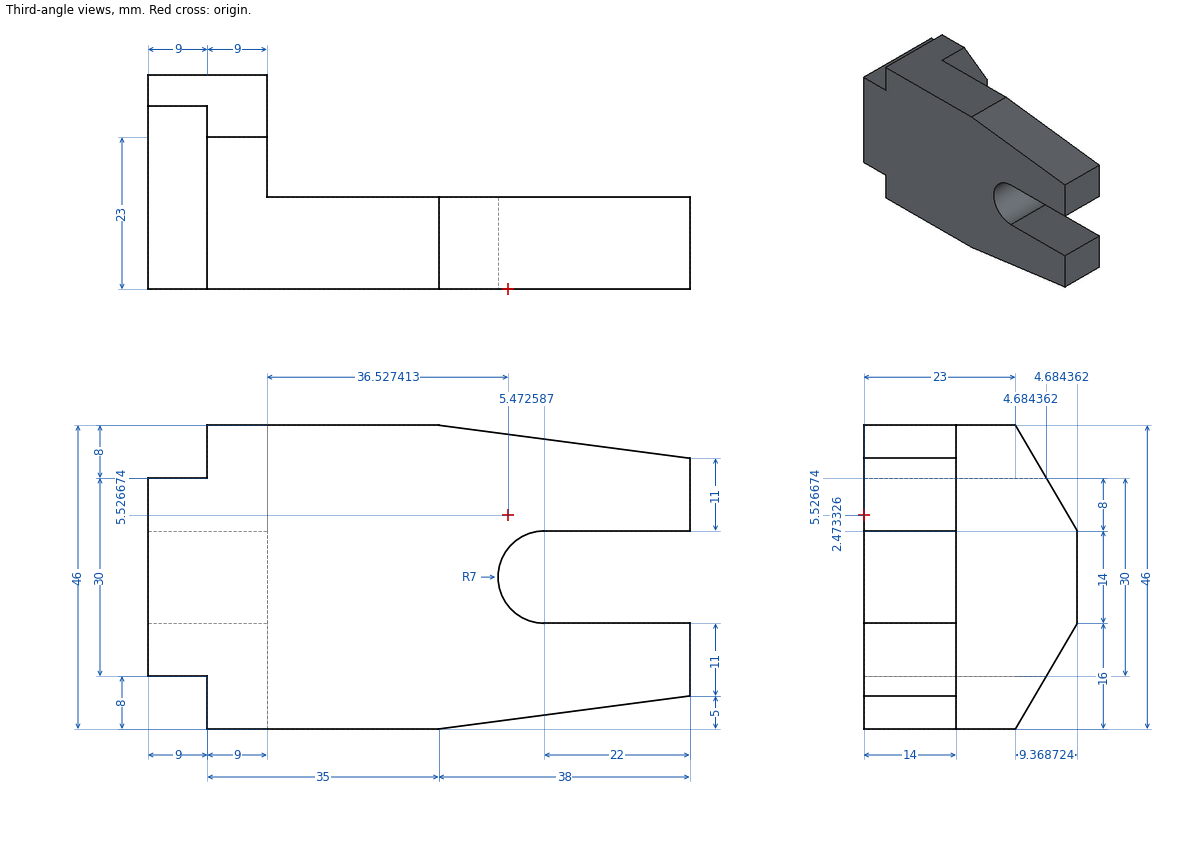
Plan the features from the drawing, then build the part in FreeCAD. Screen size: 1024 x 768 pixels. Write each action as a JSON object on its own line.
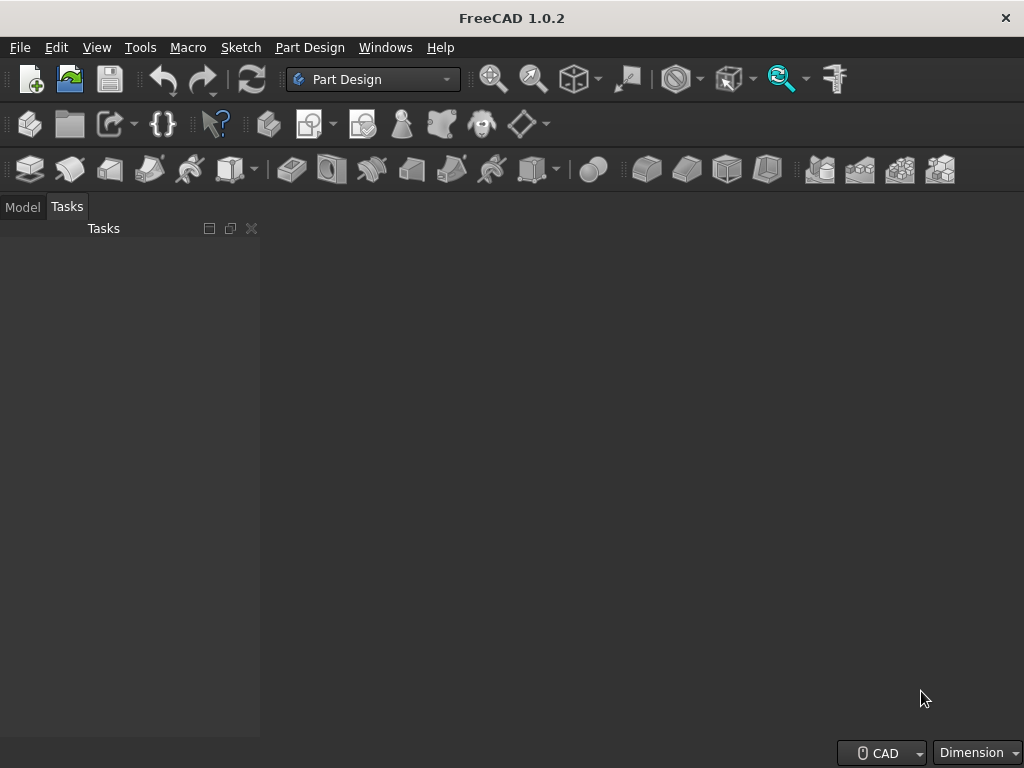
{"action": "left_click", "coordinate": [30, 80]}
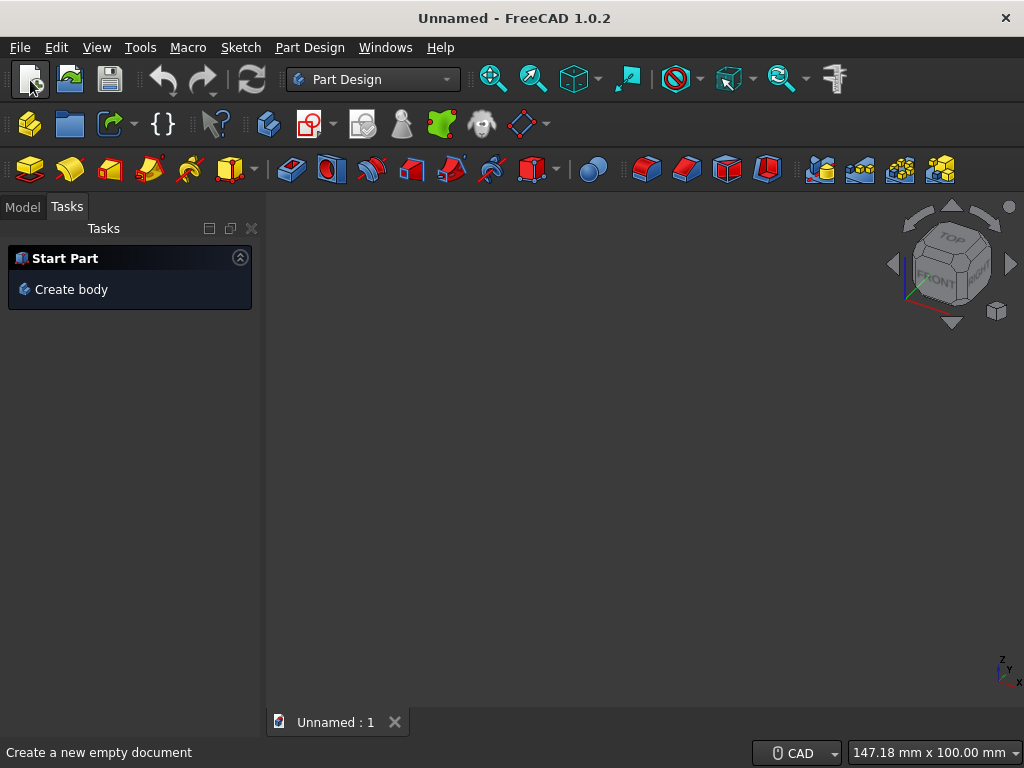
{"action": "left_click", "coordinate": [310, 124]}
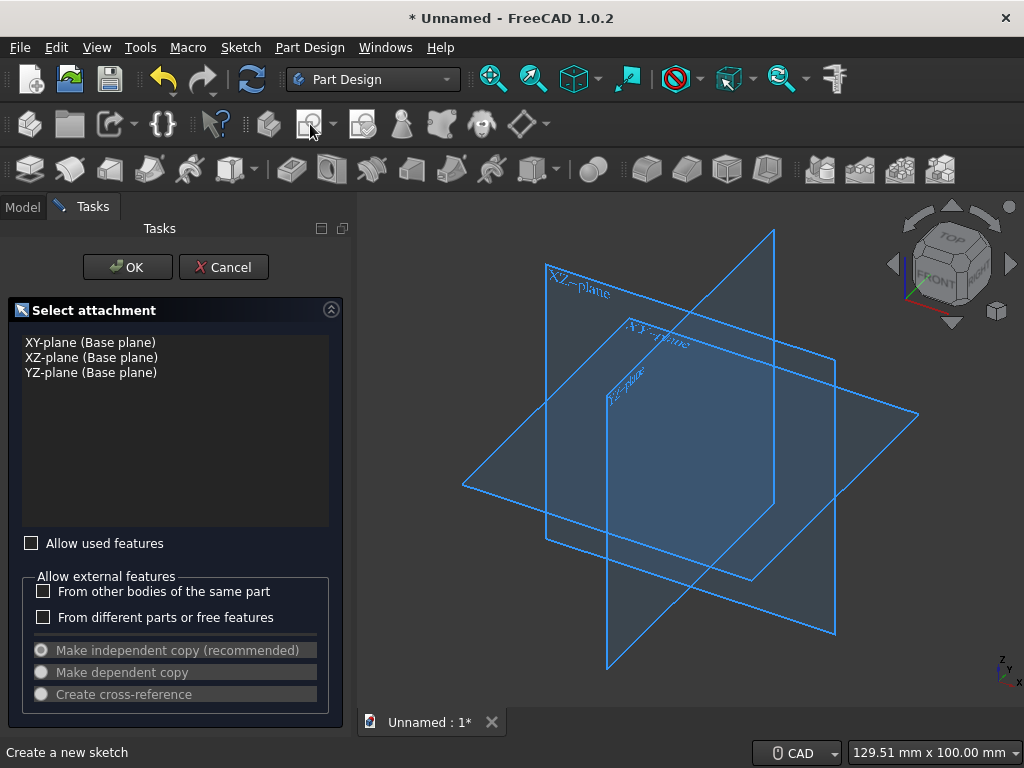
{"action": "left_click", "coordinate": [82, 358]}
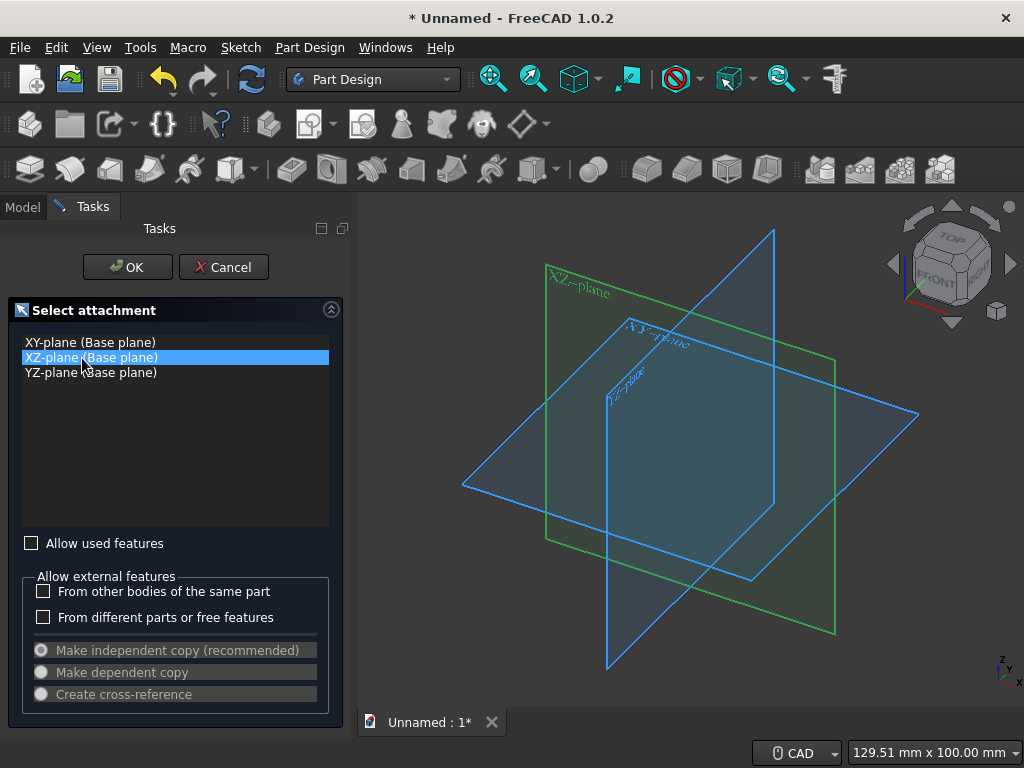
{"action": "left_click", "coordinate": [128, 267]}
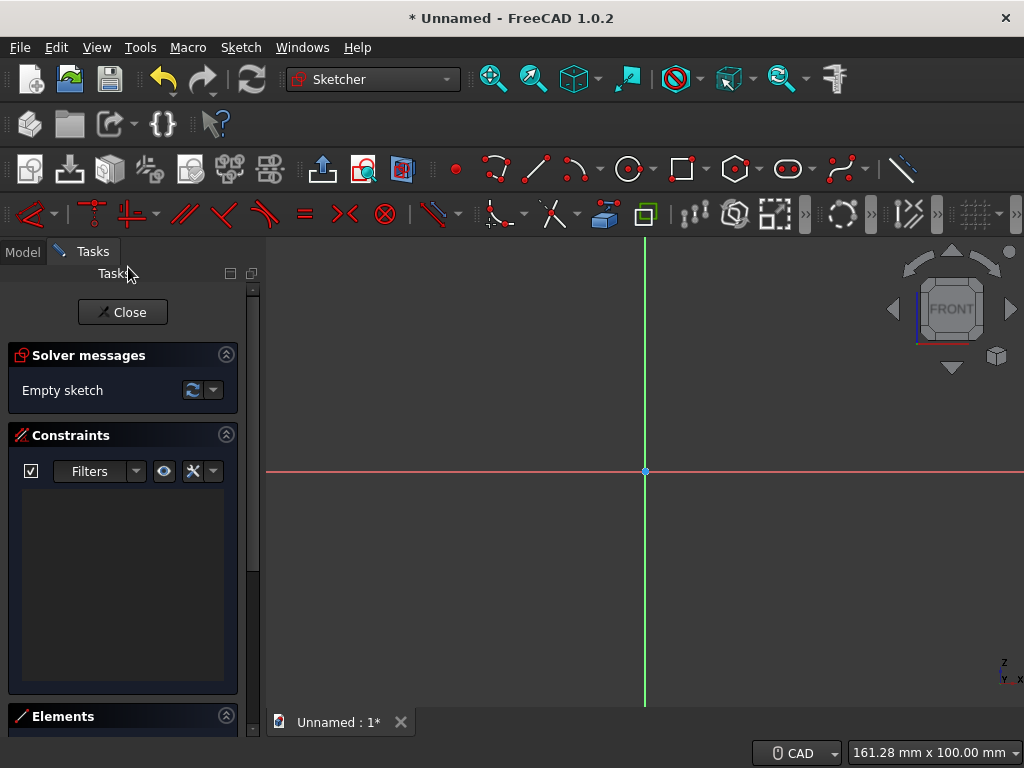
{"action": "left_click", "coordinate": [496, 170]}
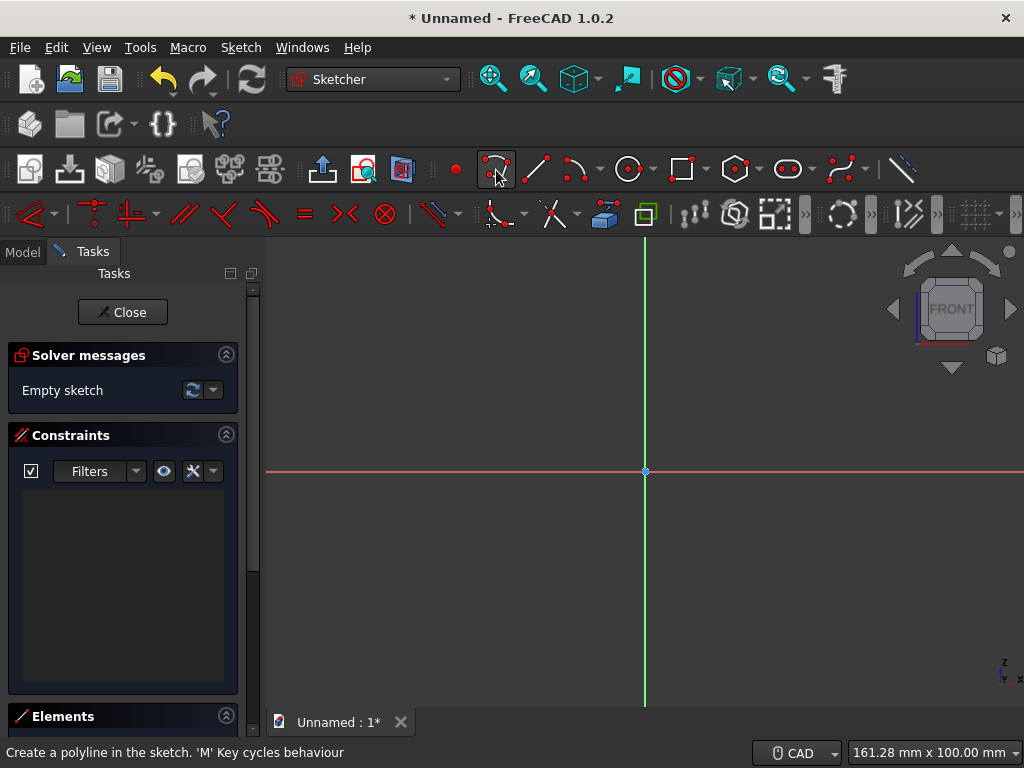
{"action": "left_click", "coordinate": [671, 549]}
{"action": "left_click", "coordinate": [774, 549]}
{"action": "left_click", "coordinate": [774, 601]}
{"action": "left_click", "coordinate": [596, 625]}
{"action": "left_click", "coordinate": [431, 625]}
{"action": "left_click", "coordinate": [431, 587]}
{"action": "left_click", "coordinate": [389, 587]}
{"action": "left_click", "coordinate": [389, 446]}
{"action": "left_click", "coordinate": [431, 446]}
{"action": "left_click", "coordinate": [431, 408]}
{"action": "left_click", "coordinate": [596, 408]}
{"action": "left_click", "coordinate": [774, 432]}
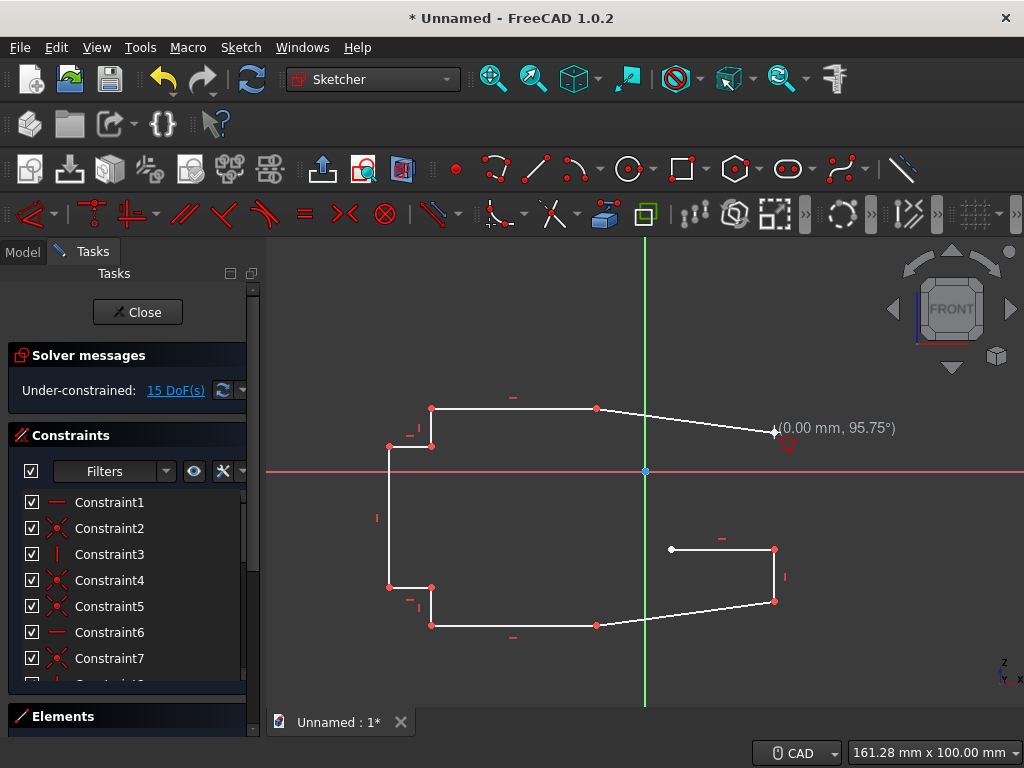
{"action": "scroll", "coordinate": [774, 484], "scroll_direction": "up", "scroll_amount": 2}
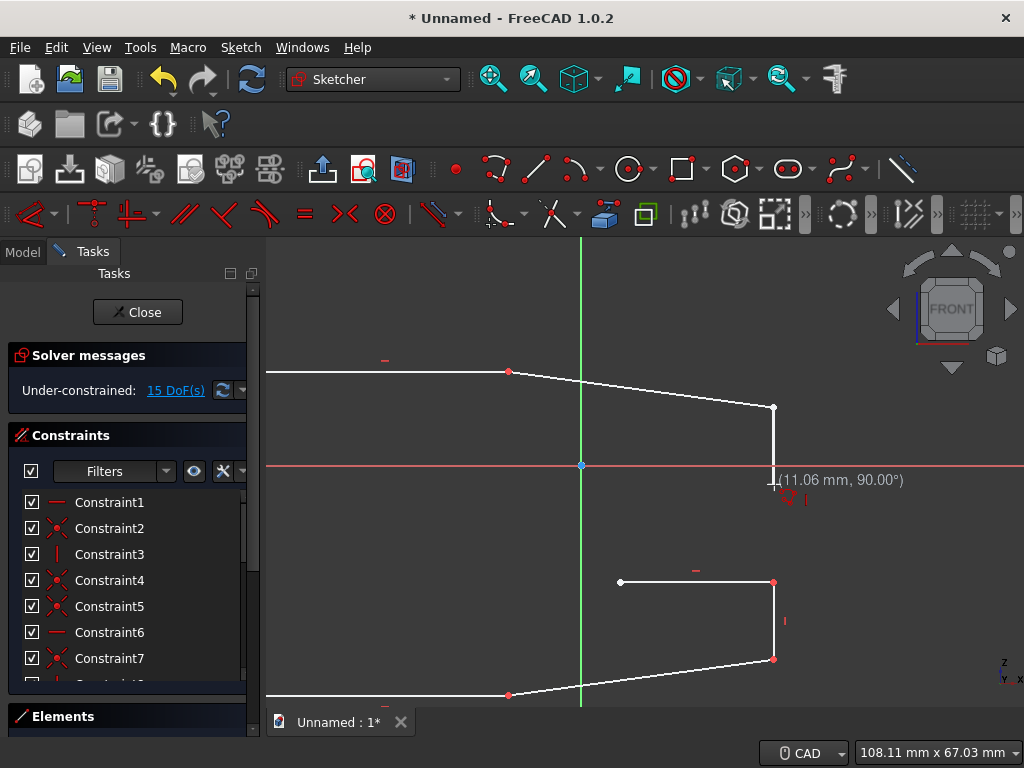
{"action": "left_click", "coordinate": [774, 483]}
{"action": "left_click", "coordinate": [620, 483]}
{"action": "right_click", "coordinate": [620, 483]}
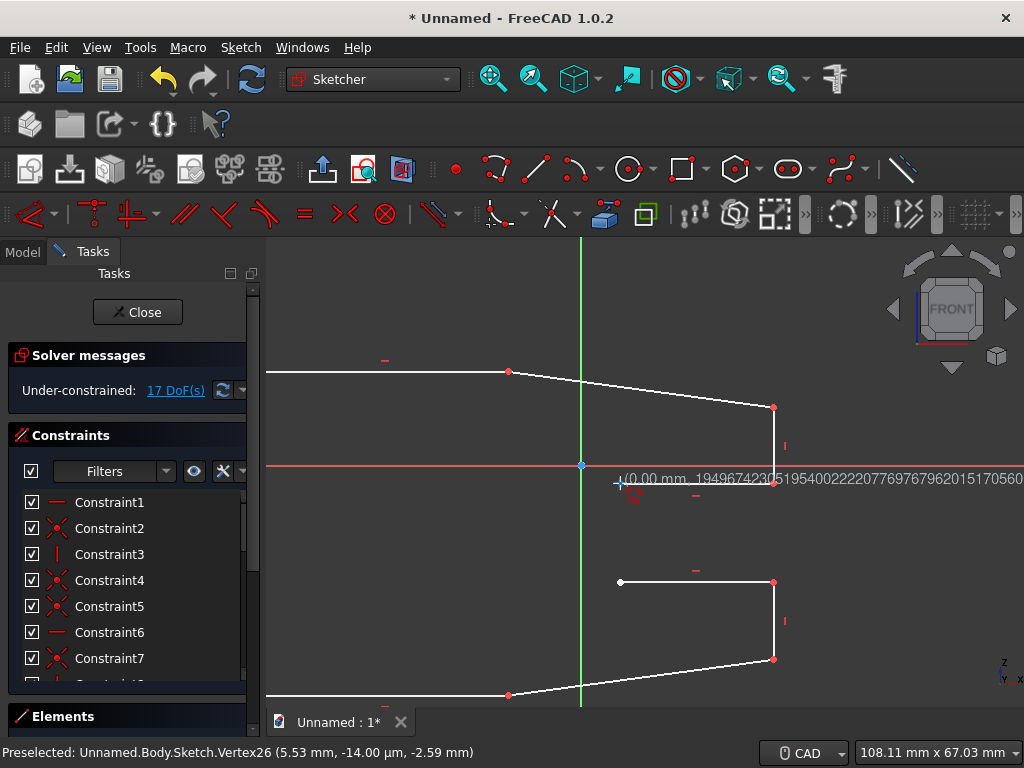
{"action": "left_click", "coordinate": [602, 170]}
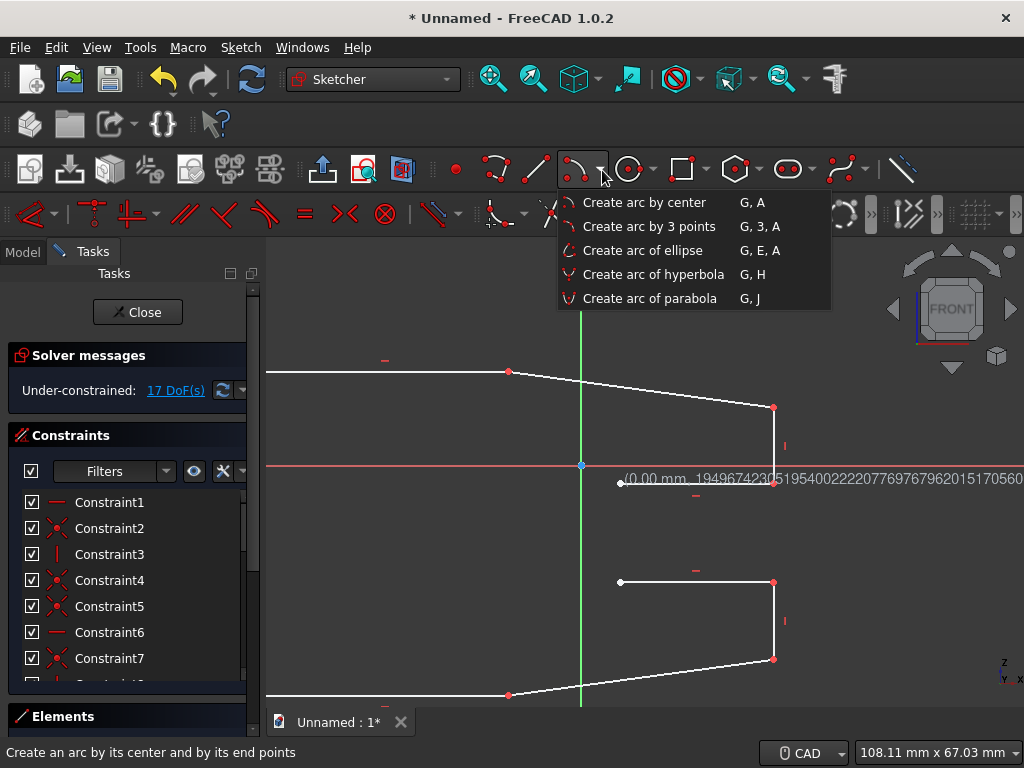
{"action": "left_click", "coordinate": [694, 226]}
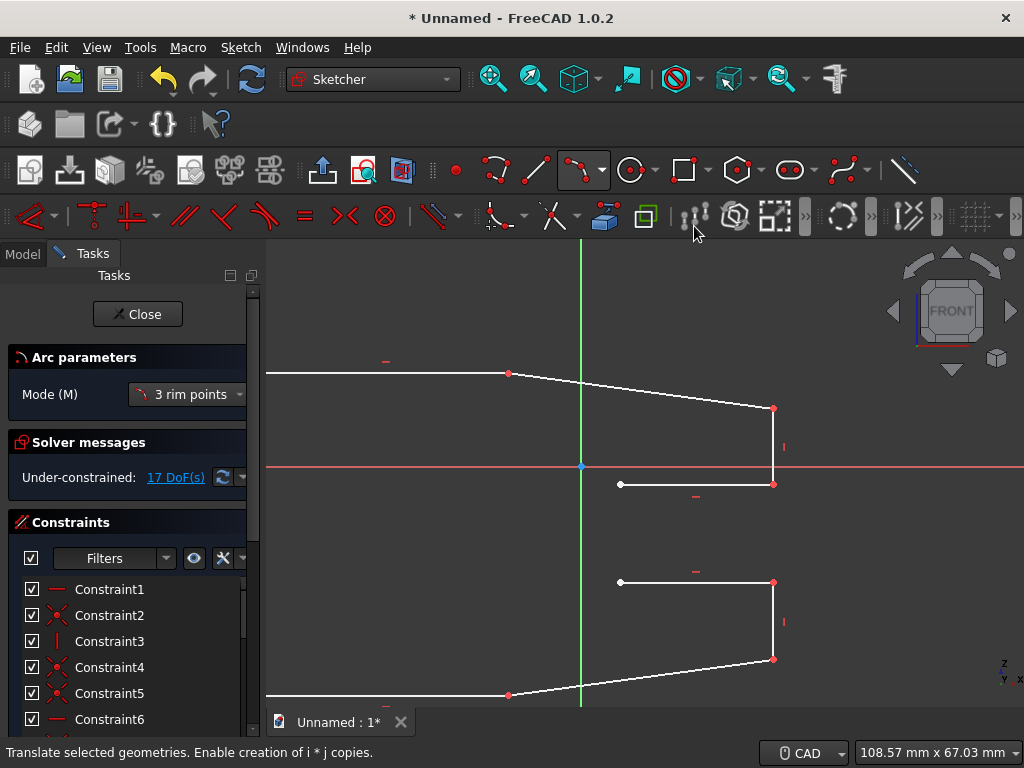
{"action": "left_click", "coordinate": [620, 485]}
{"action": "left_click", "coordinate": [620, 583]}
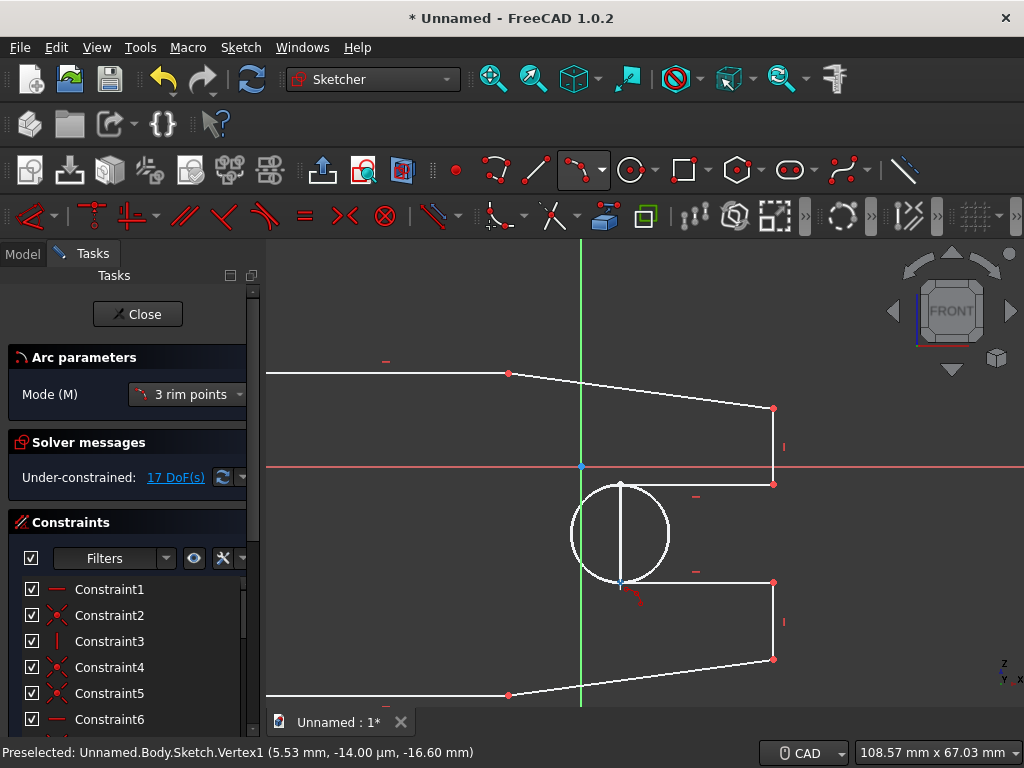
{"action": "scroll", "coordinate": [571, 533], "scroll_direction": "up", "scroll_amount": 2}